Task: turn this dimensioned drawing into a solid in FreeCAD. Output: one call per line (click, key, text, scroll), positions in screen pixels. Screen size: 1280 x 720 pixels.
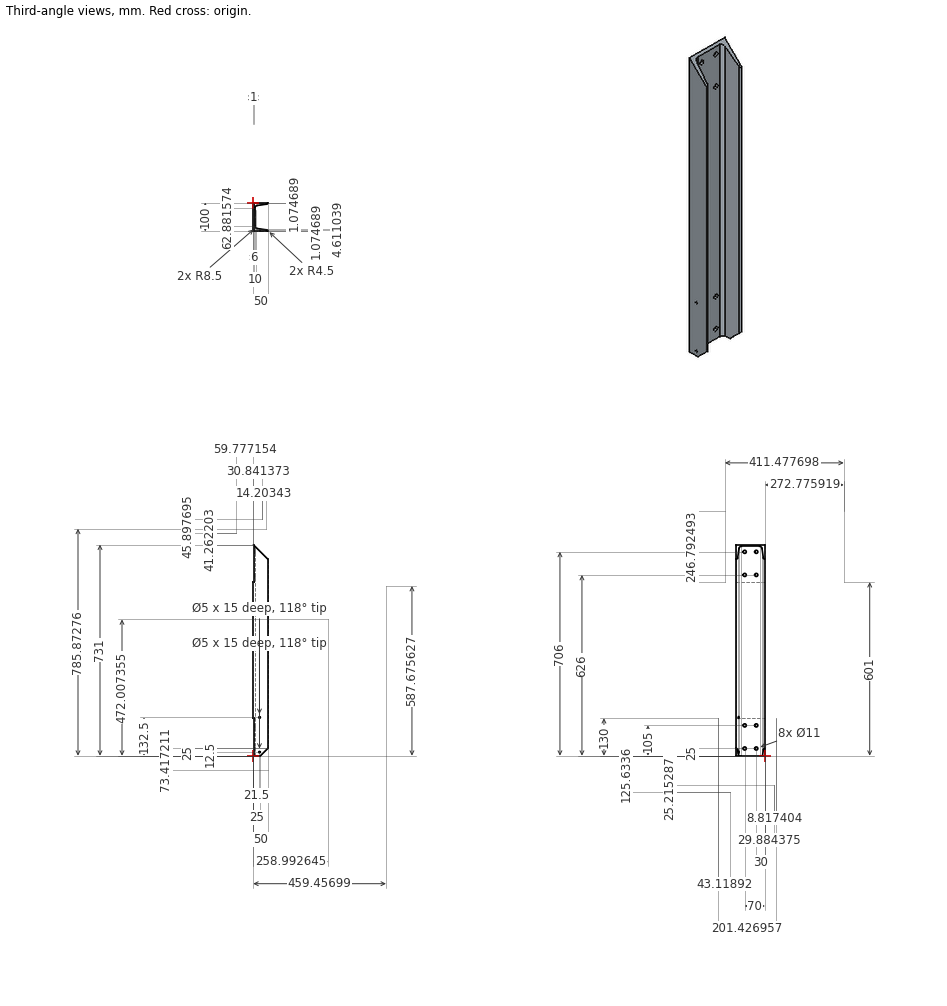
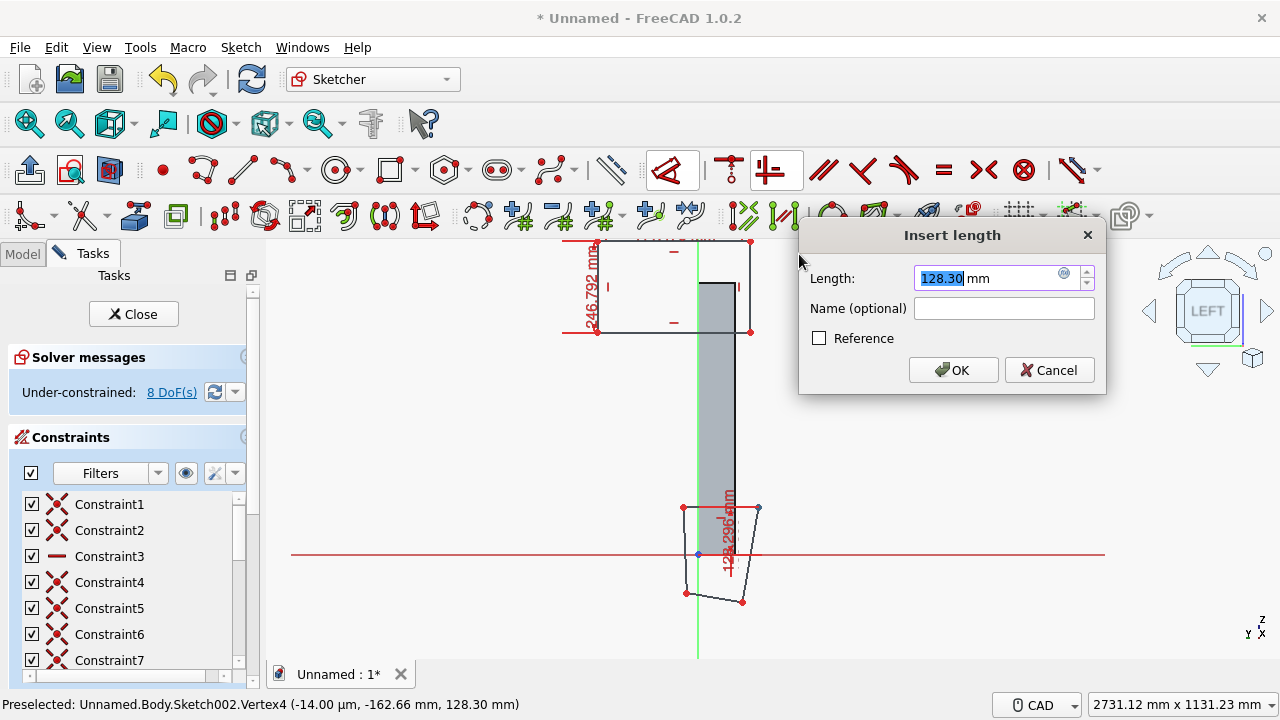
text(130)
key(Return)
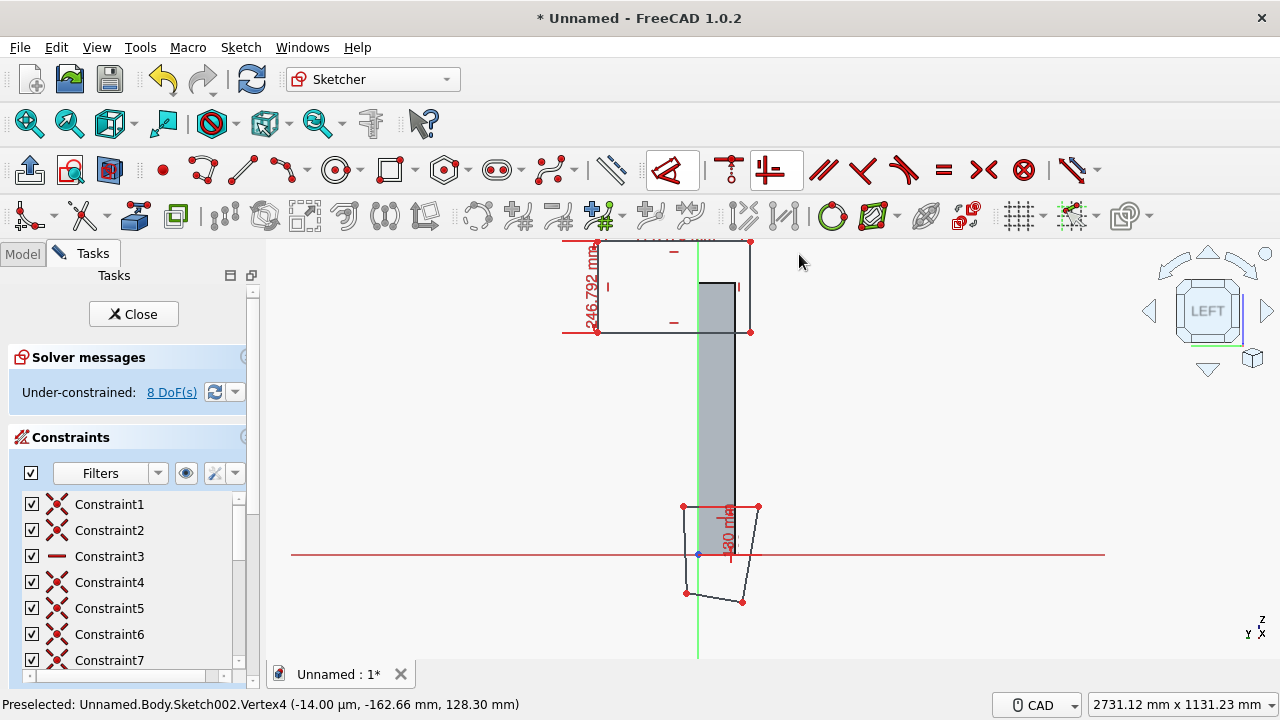
click(598, 333)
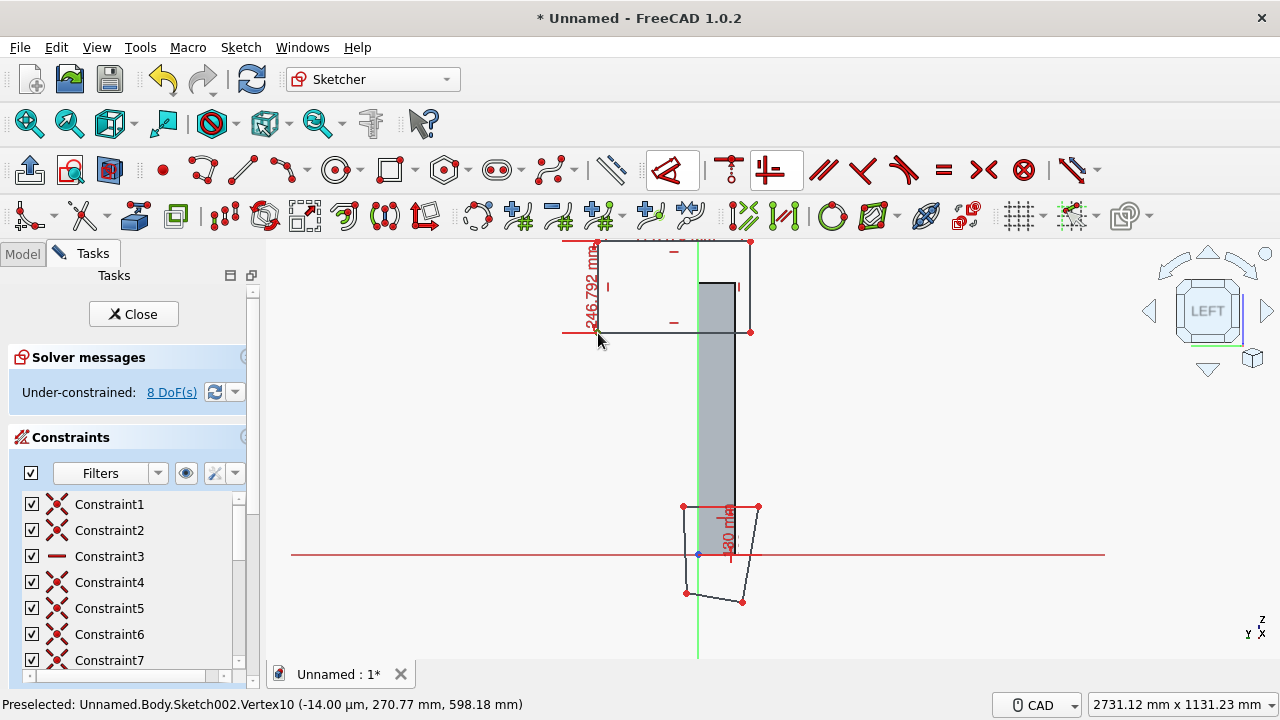
key(i)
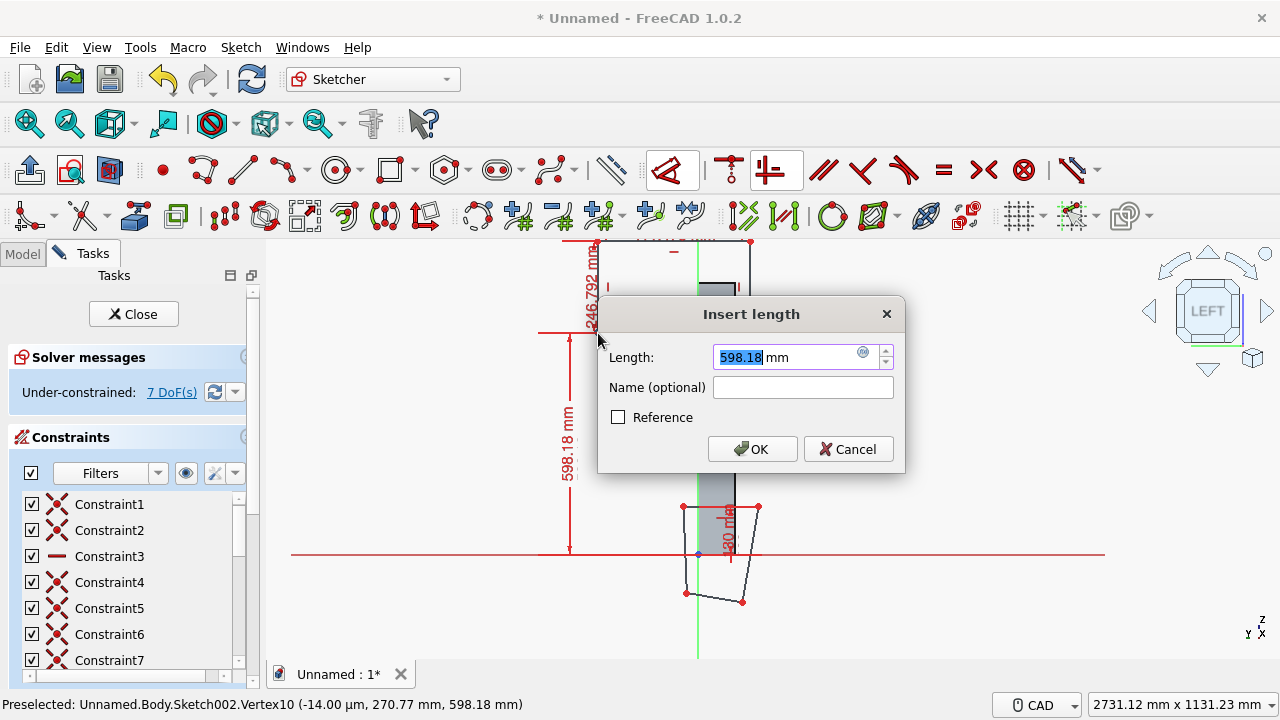
text(601)
key(Return)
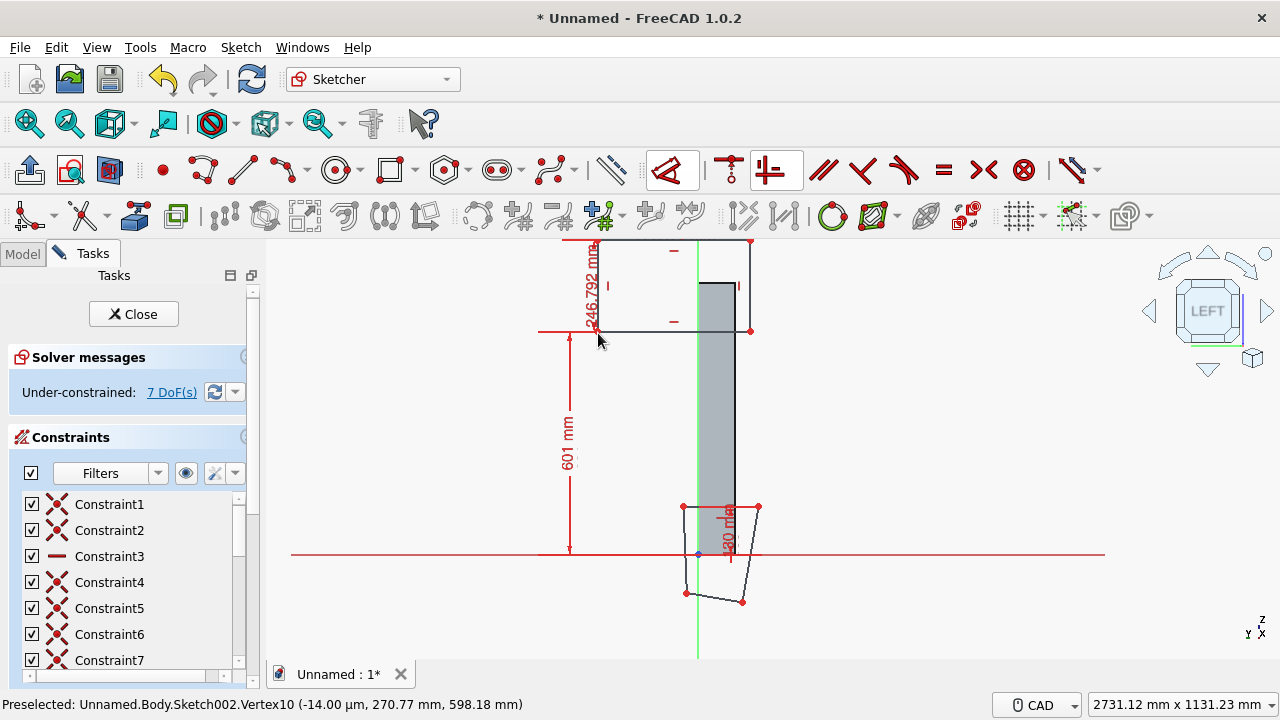
click(742, 602)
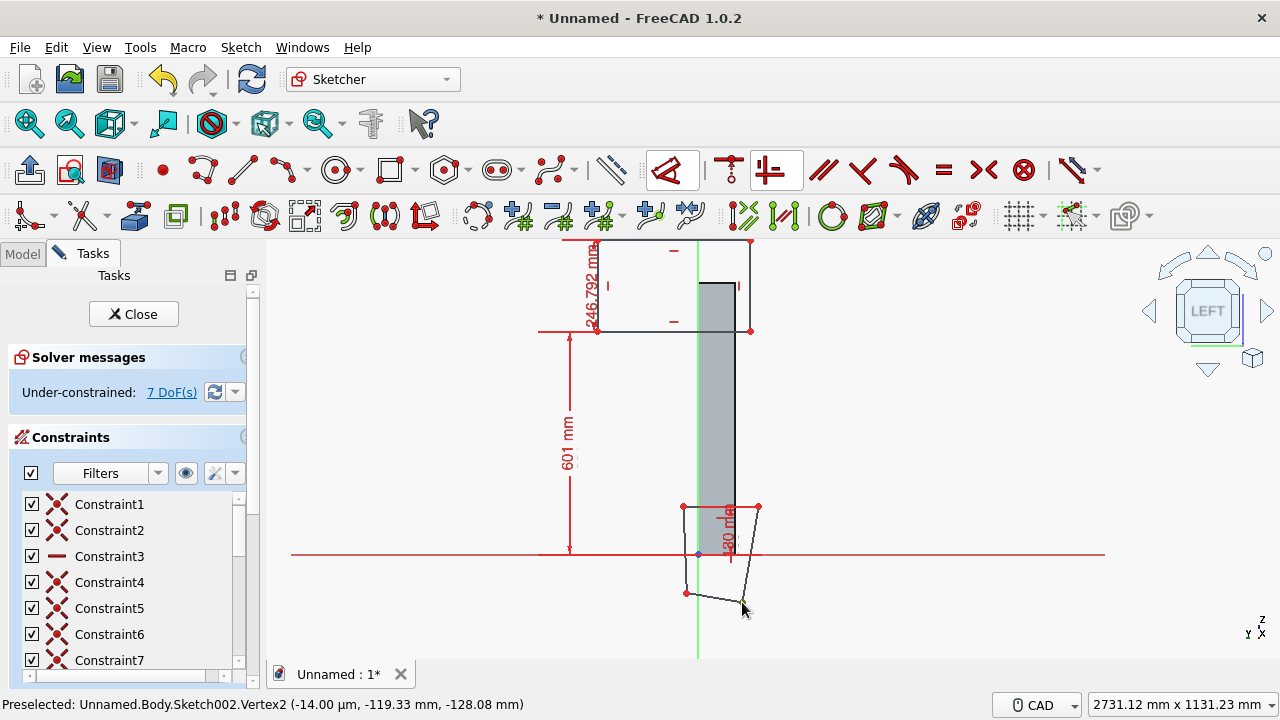
key(i)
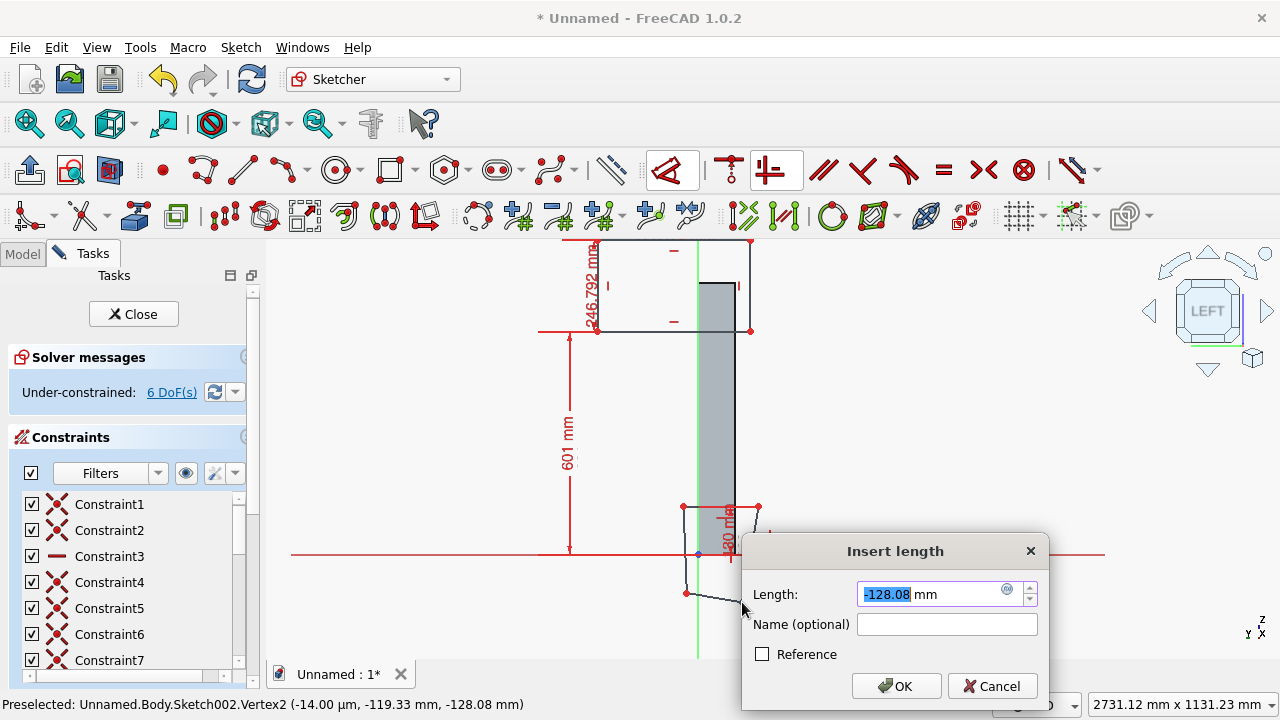
text(-125.6336)
key(Return)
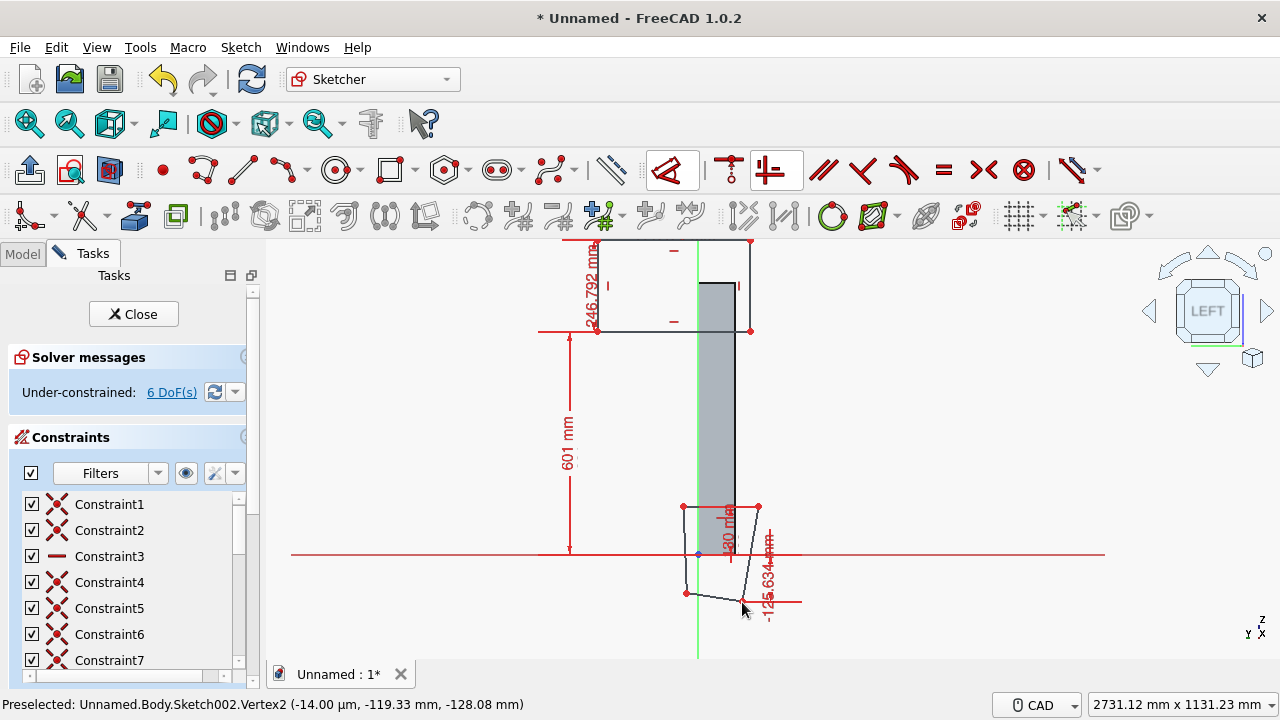
scroll(747, 573, up, 5)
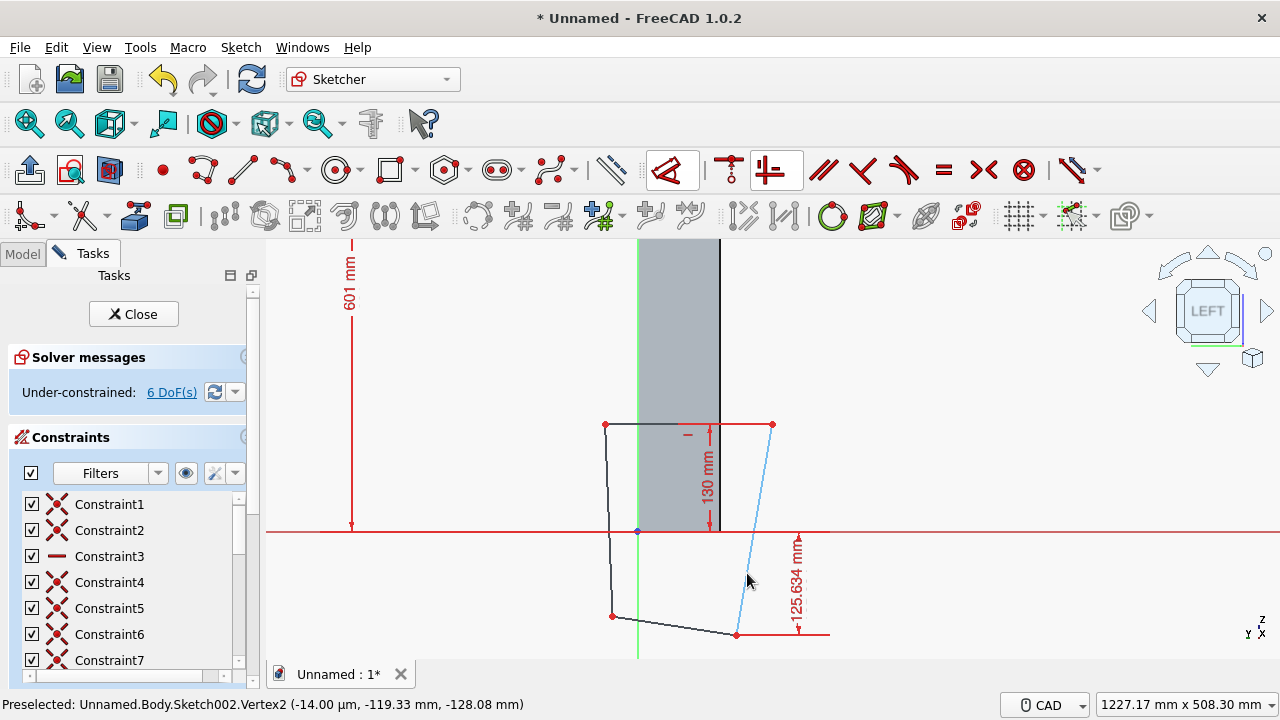
click(747, 572)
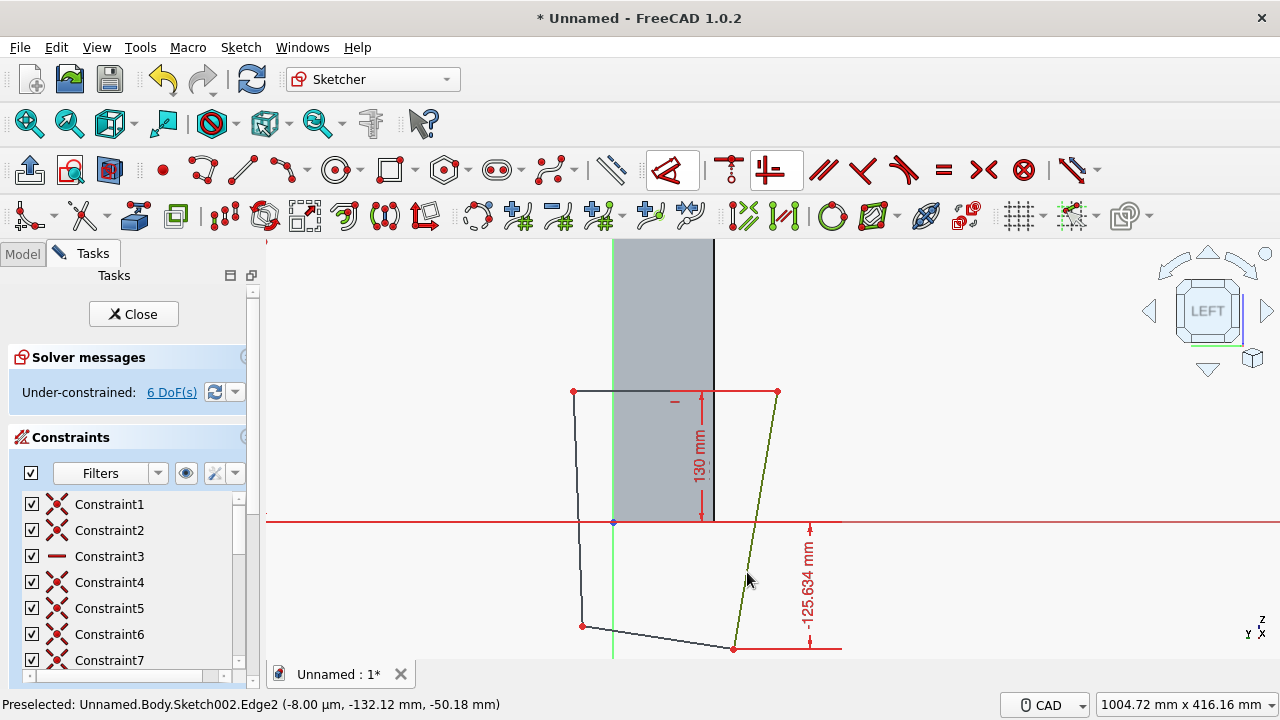
key(l)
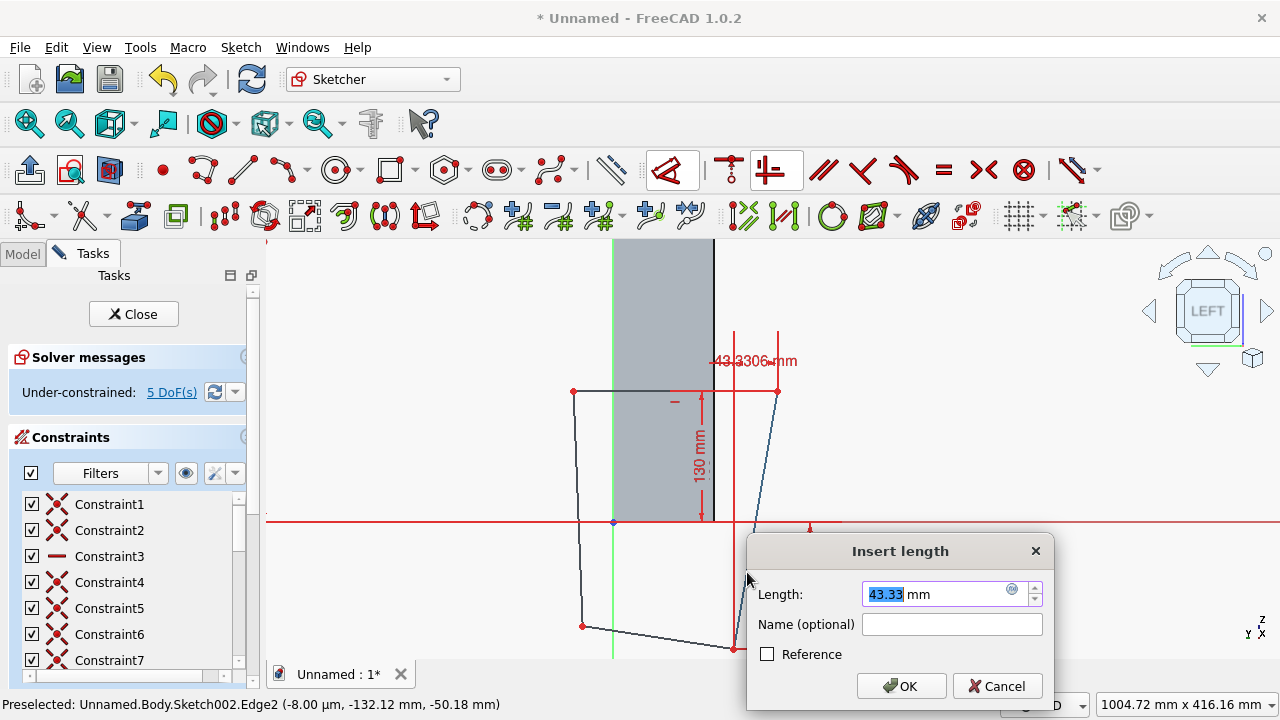
text(43.11892)
key(Return)